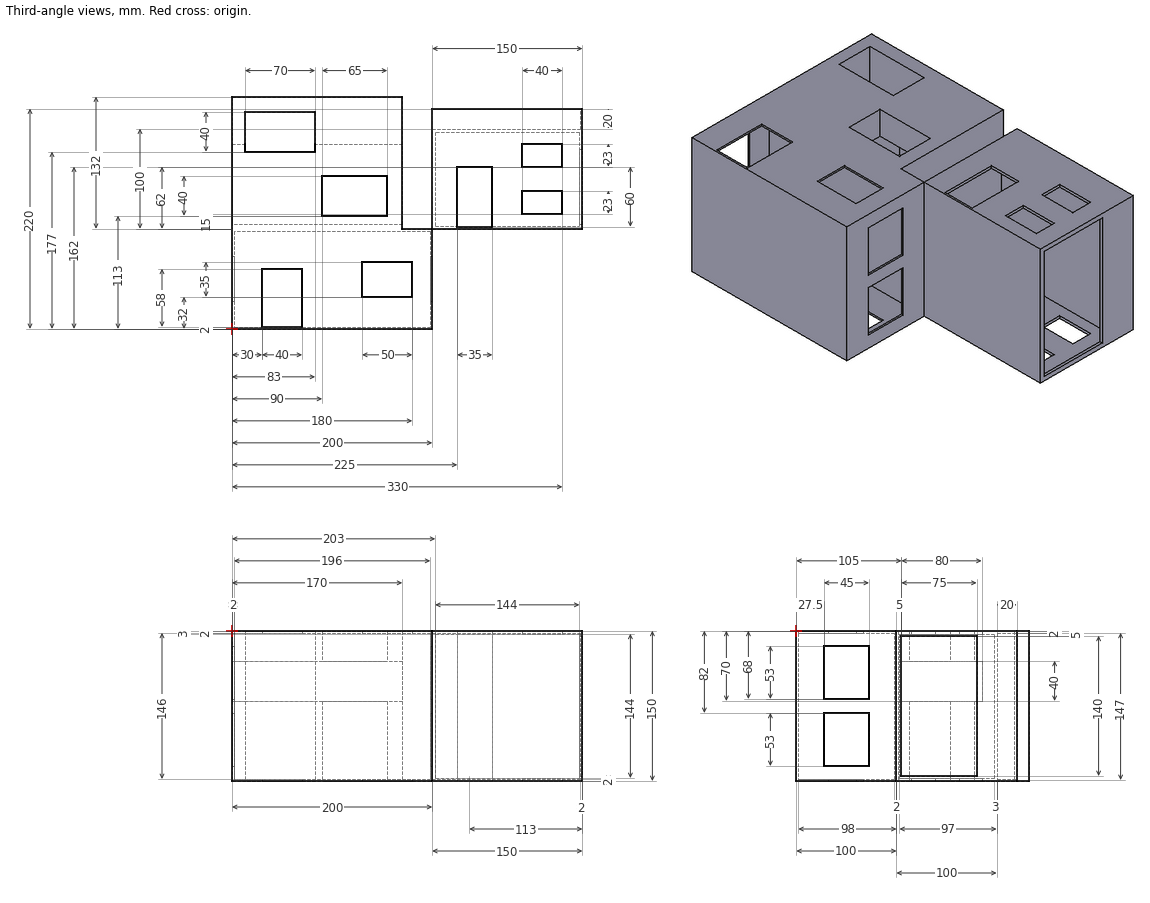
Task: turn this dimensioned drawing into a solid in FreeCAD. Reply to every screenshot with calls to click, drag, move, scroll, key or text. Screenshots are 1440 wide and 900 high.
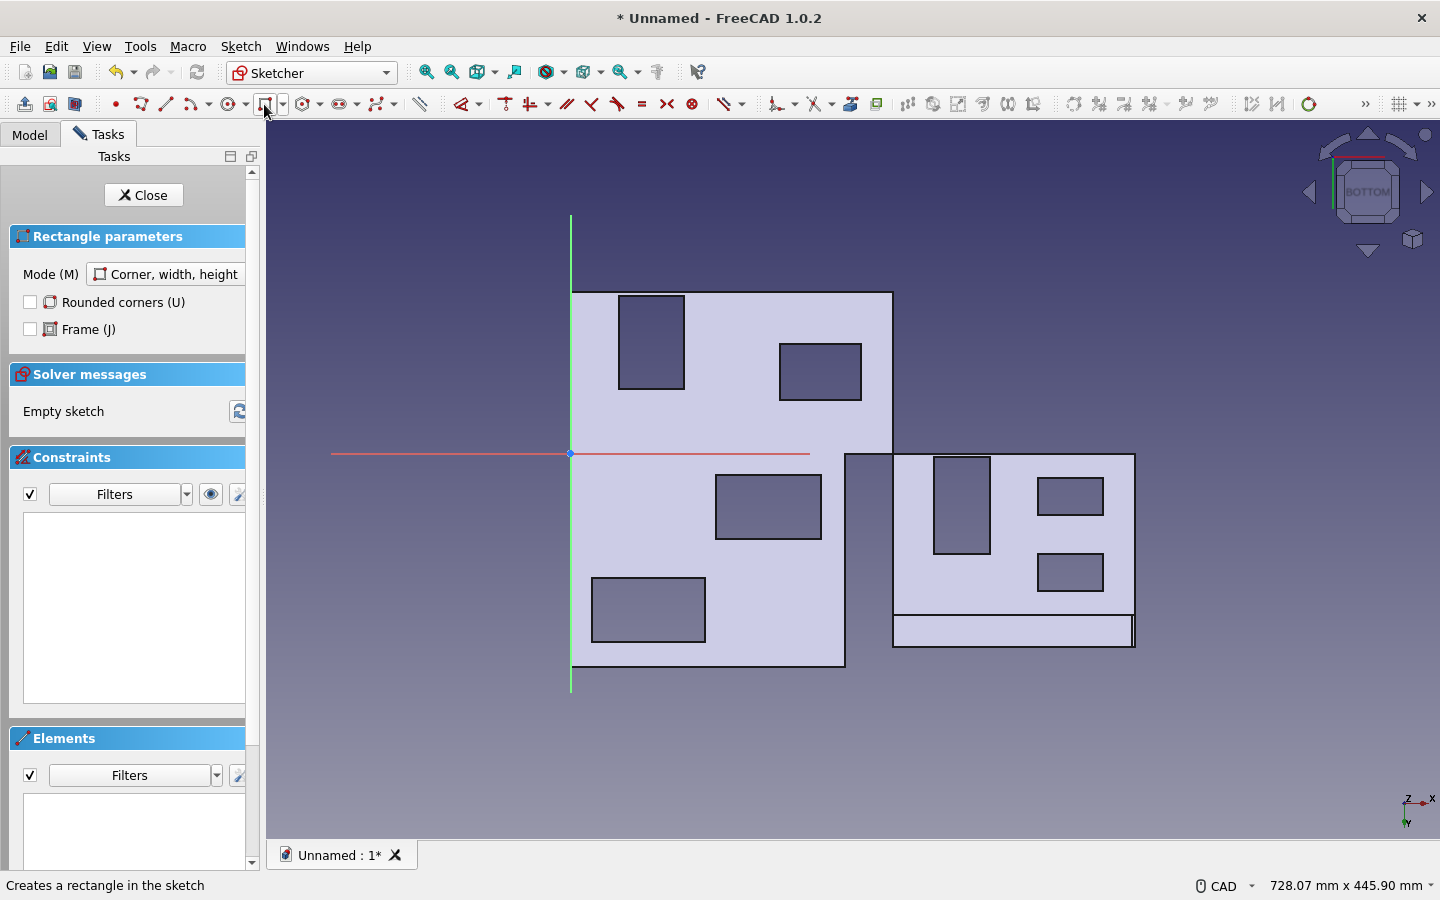
click(893, 615)
move(1135, 647)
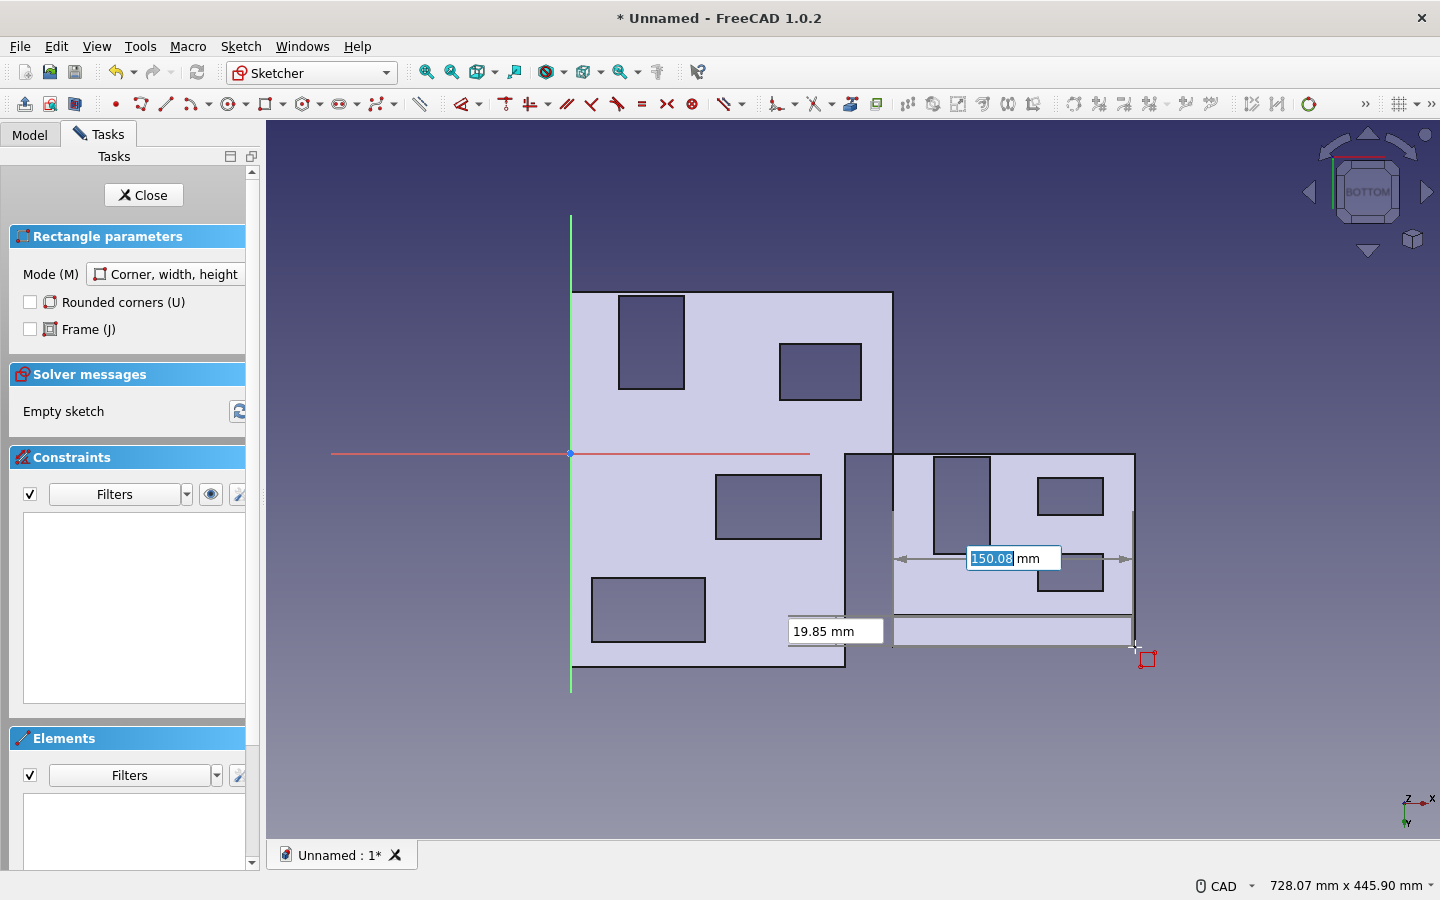
text(150)
key(Tab)
text(20)
key(Return)
key(Escape)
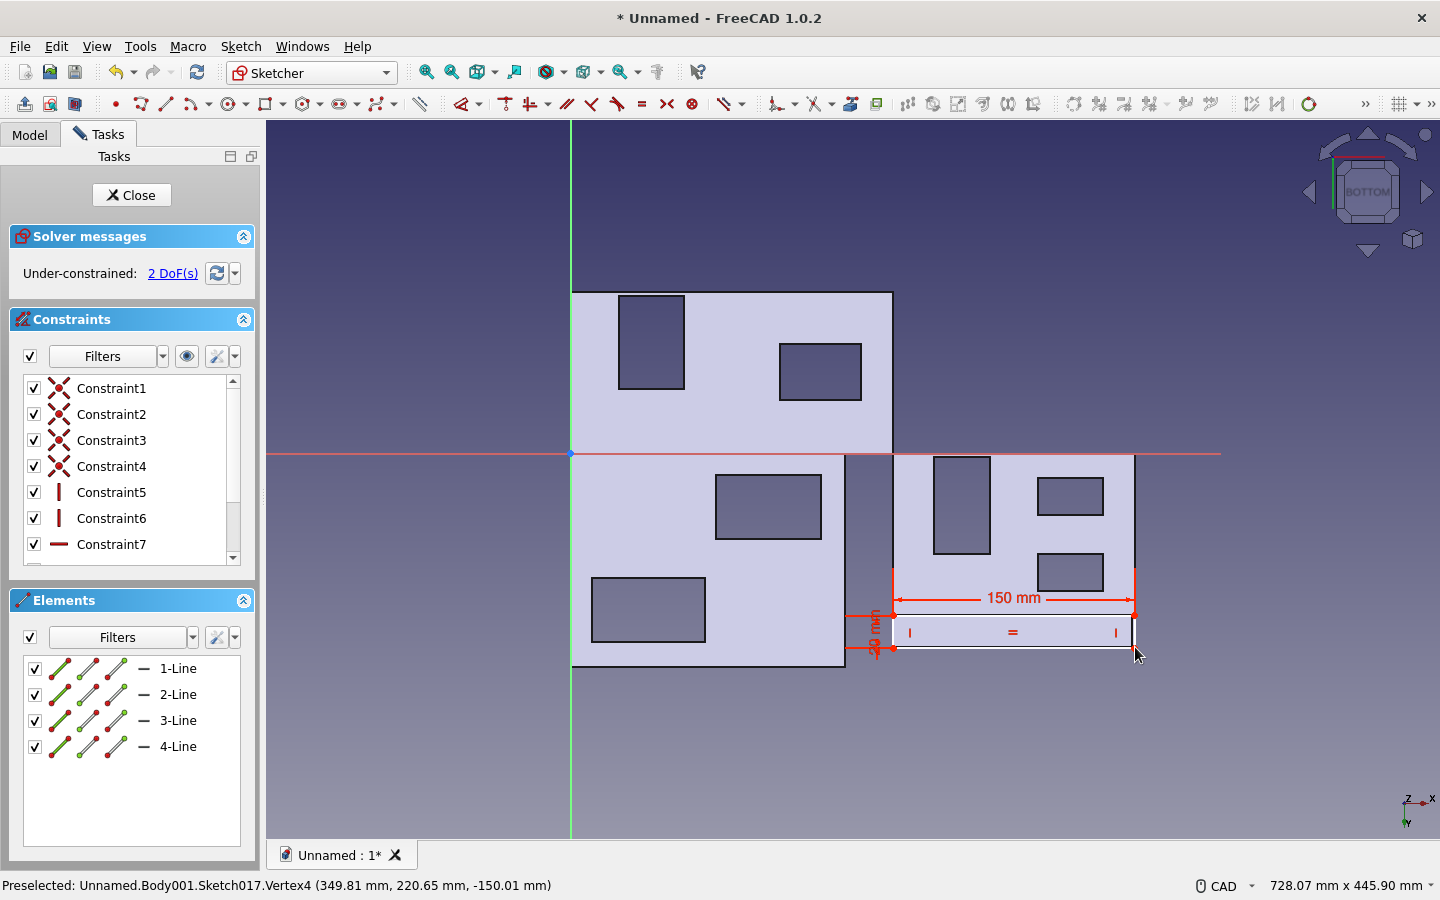
click(460, 104)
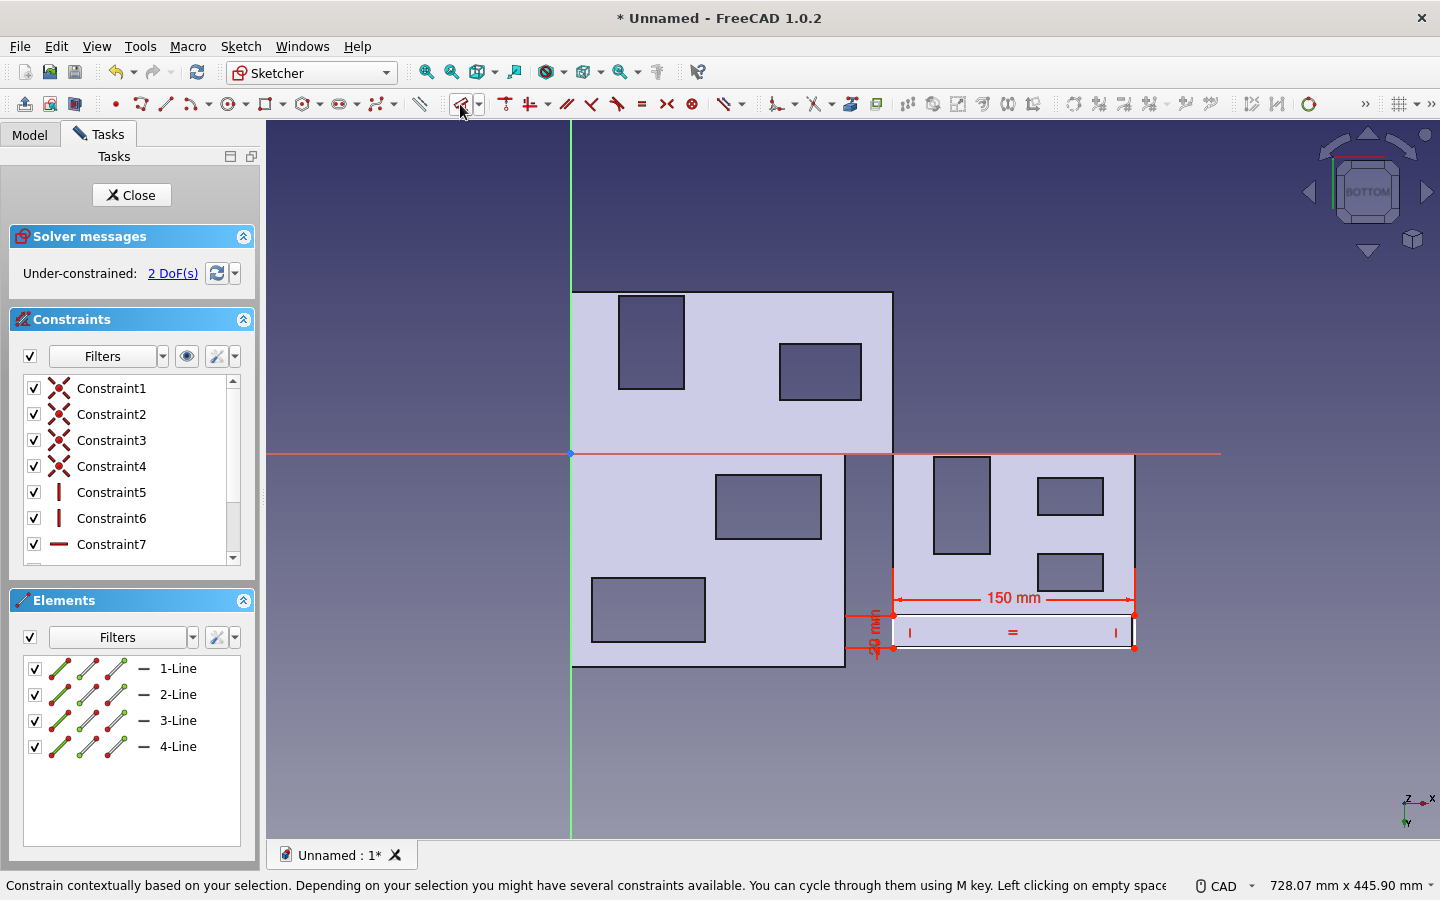
click(893, 616)
click(732, 420)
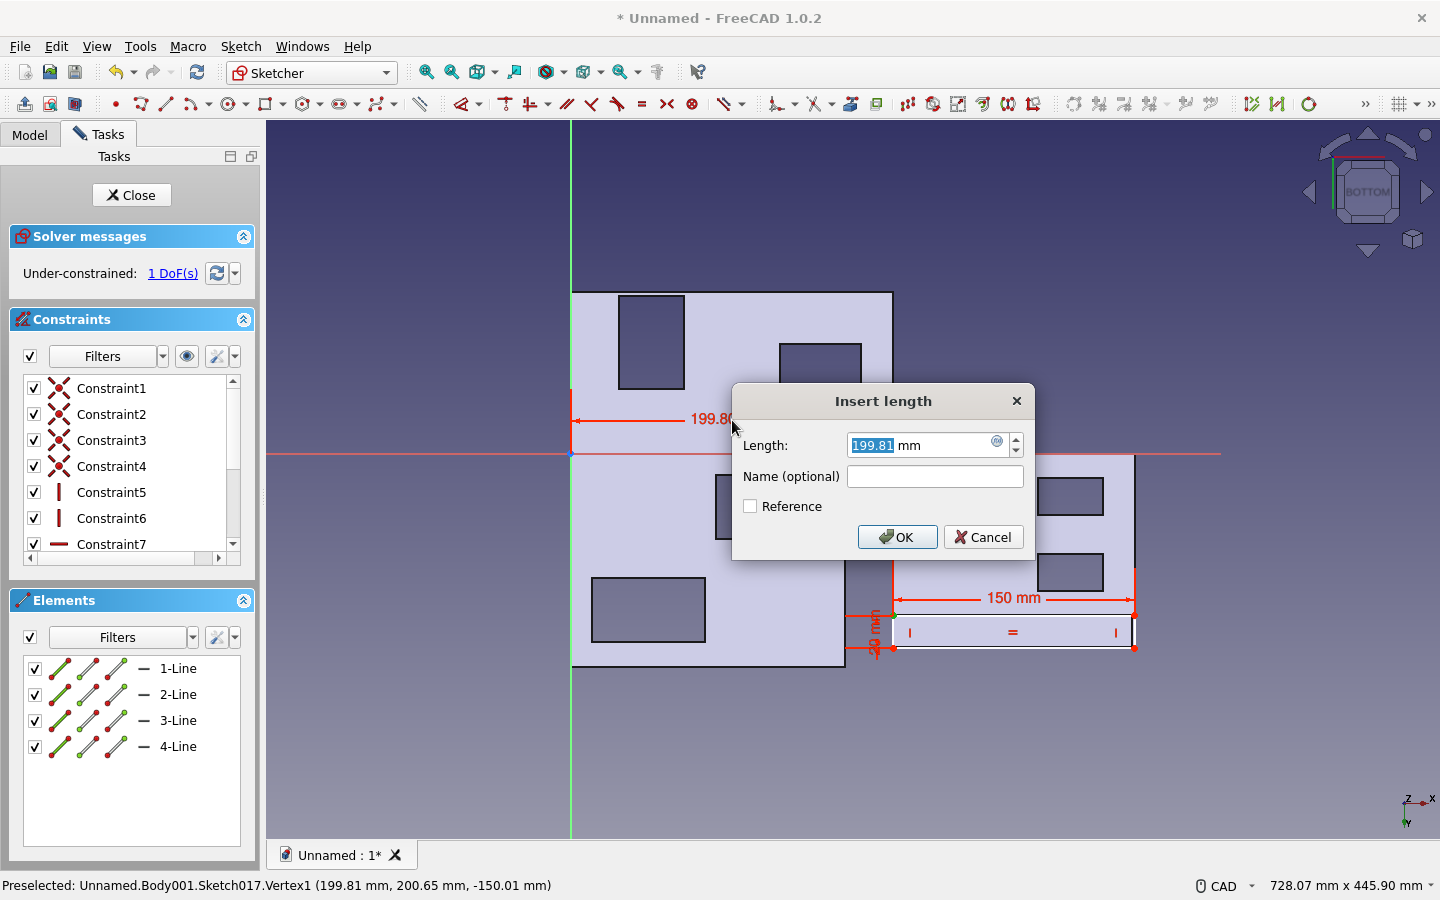
text(200)
key(Return)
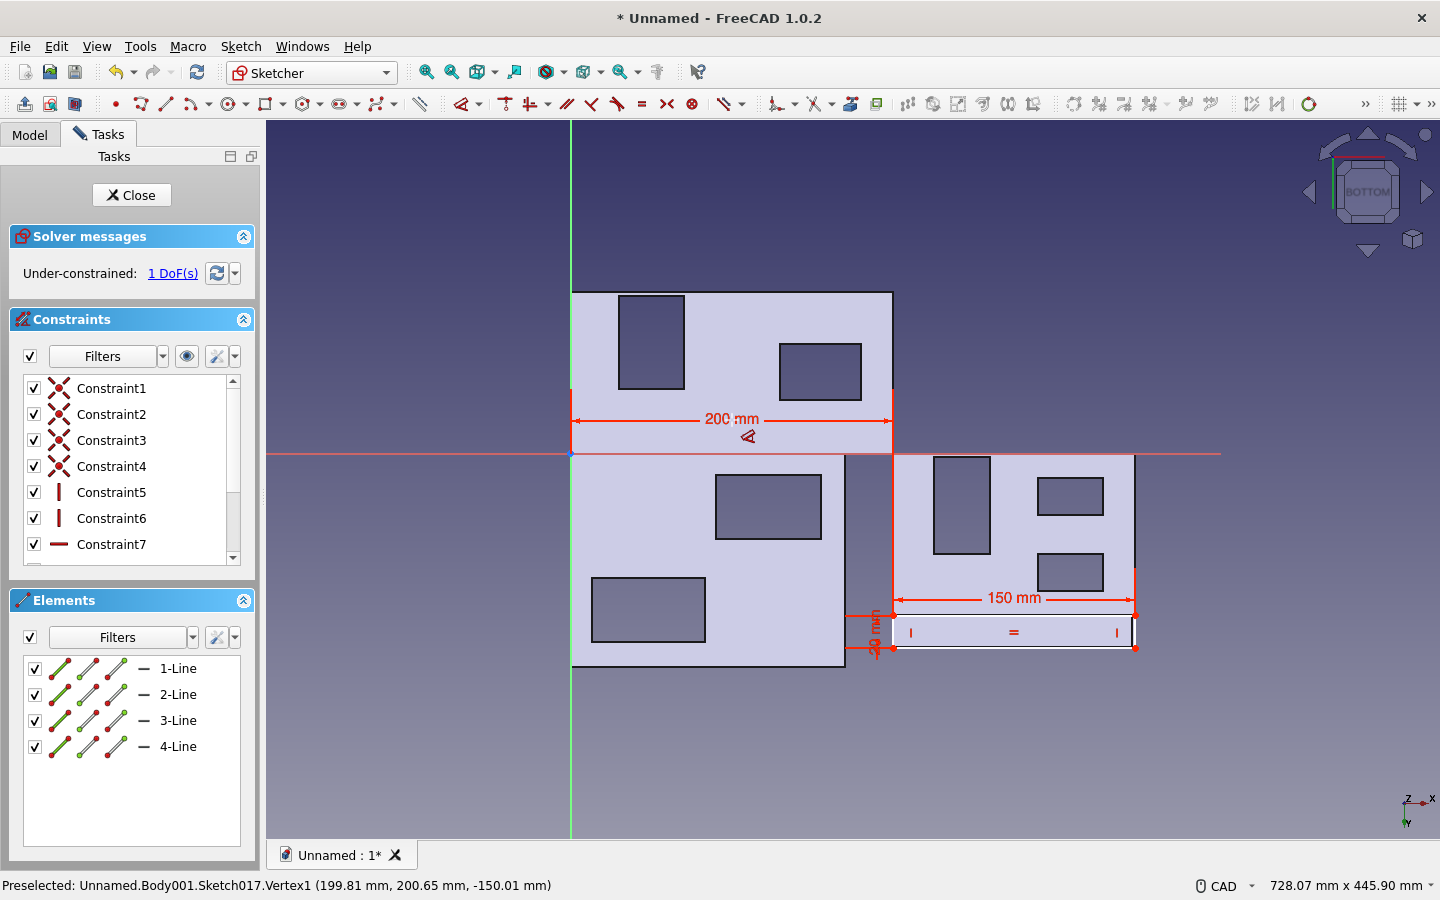
click(893, 616)
click(537, 535)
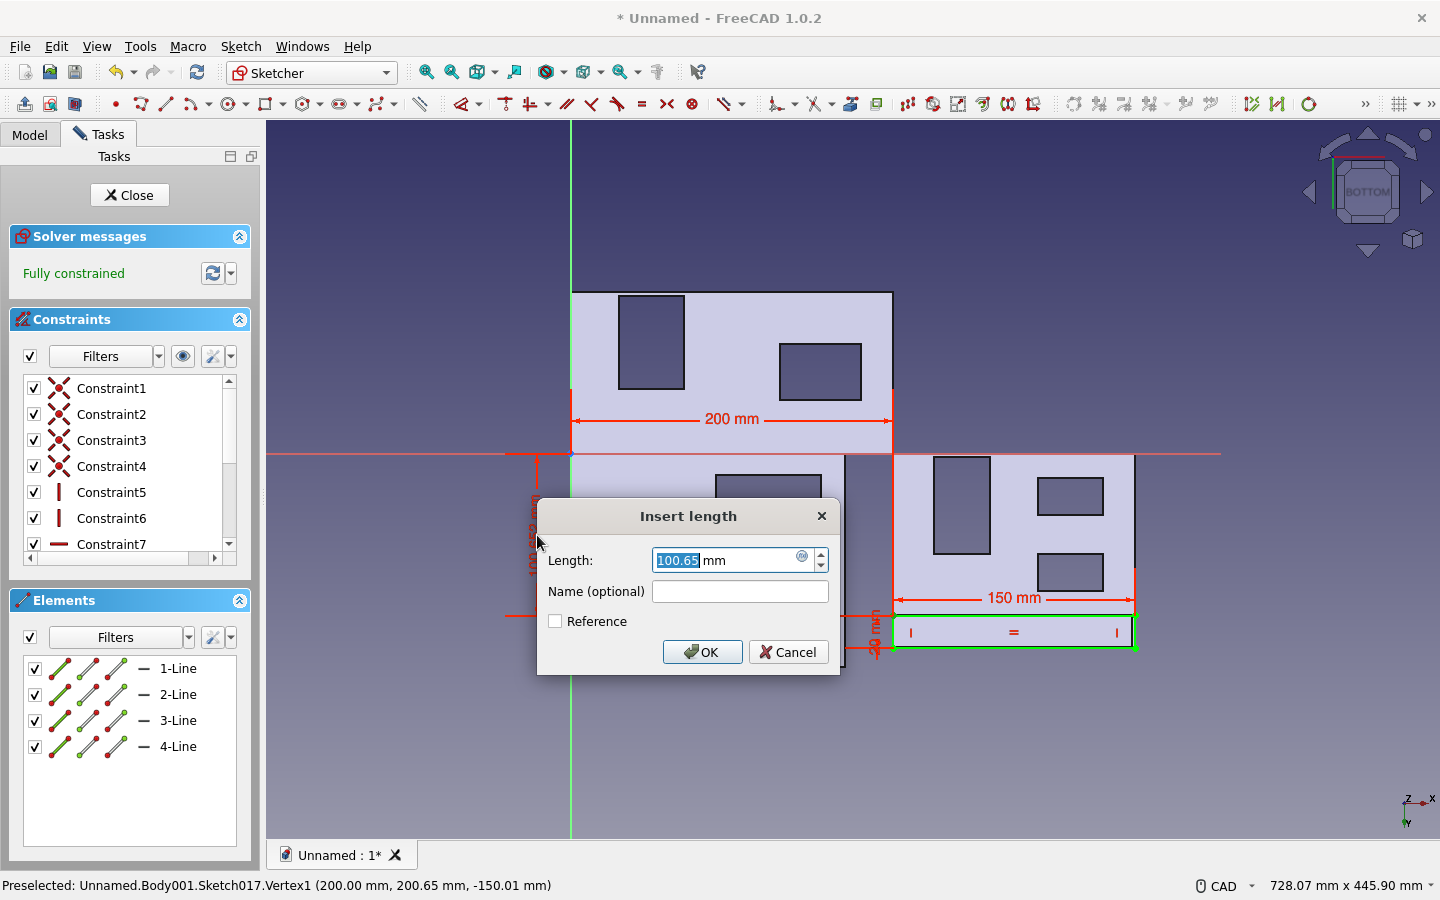
text(100)
key(Return)
key(Escape)